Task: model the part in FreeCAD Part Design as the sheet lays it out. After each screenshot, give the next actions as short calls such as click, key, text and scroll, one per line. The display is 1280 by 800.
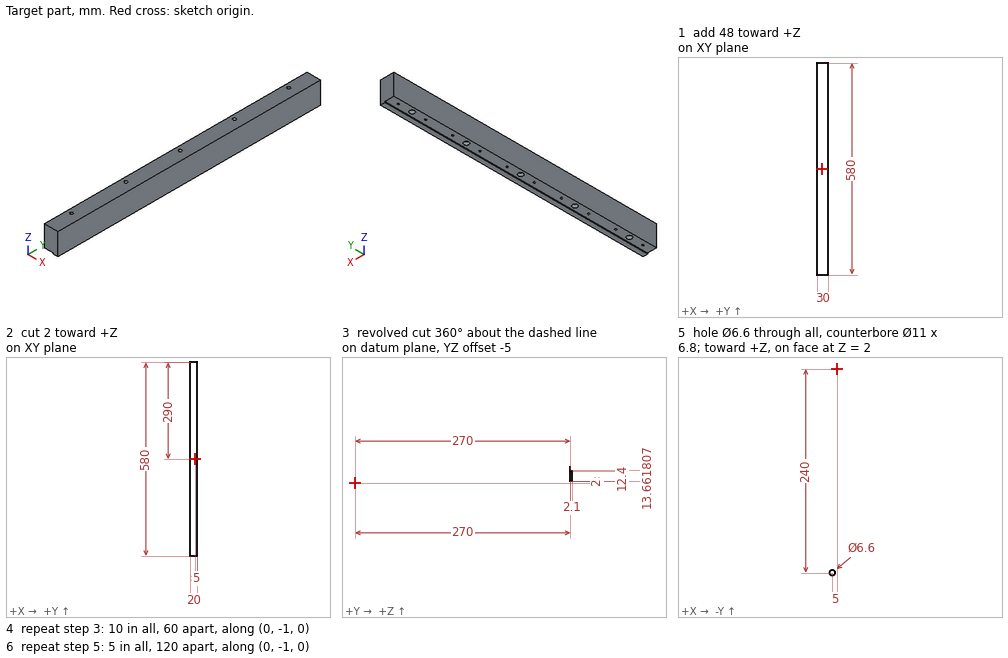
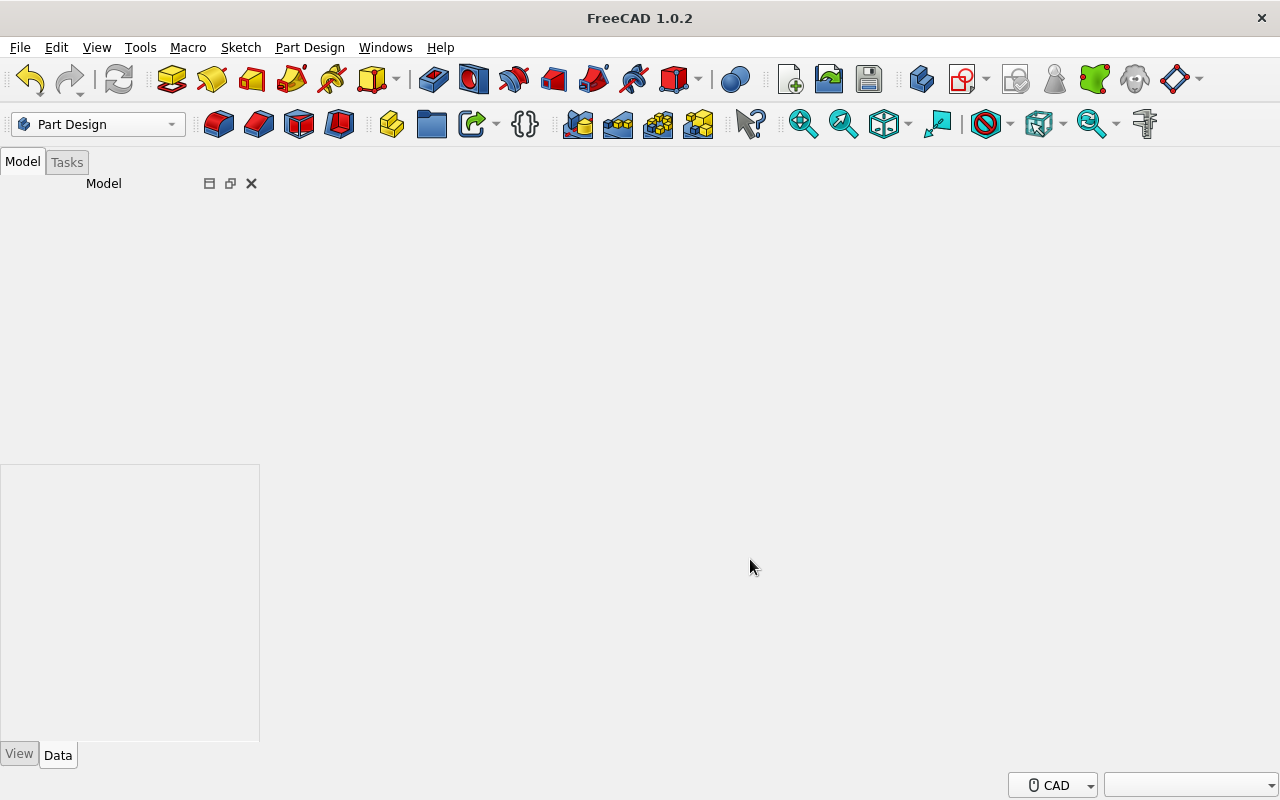
key(ctrl+n)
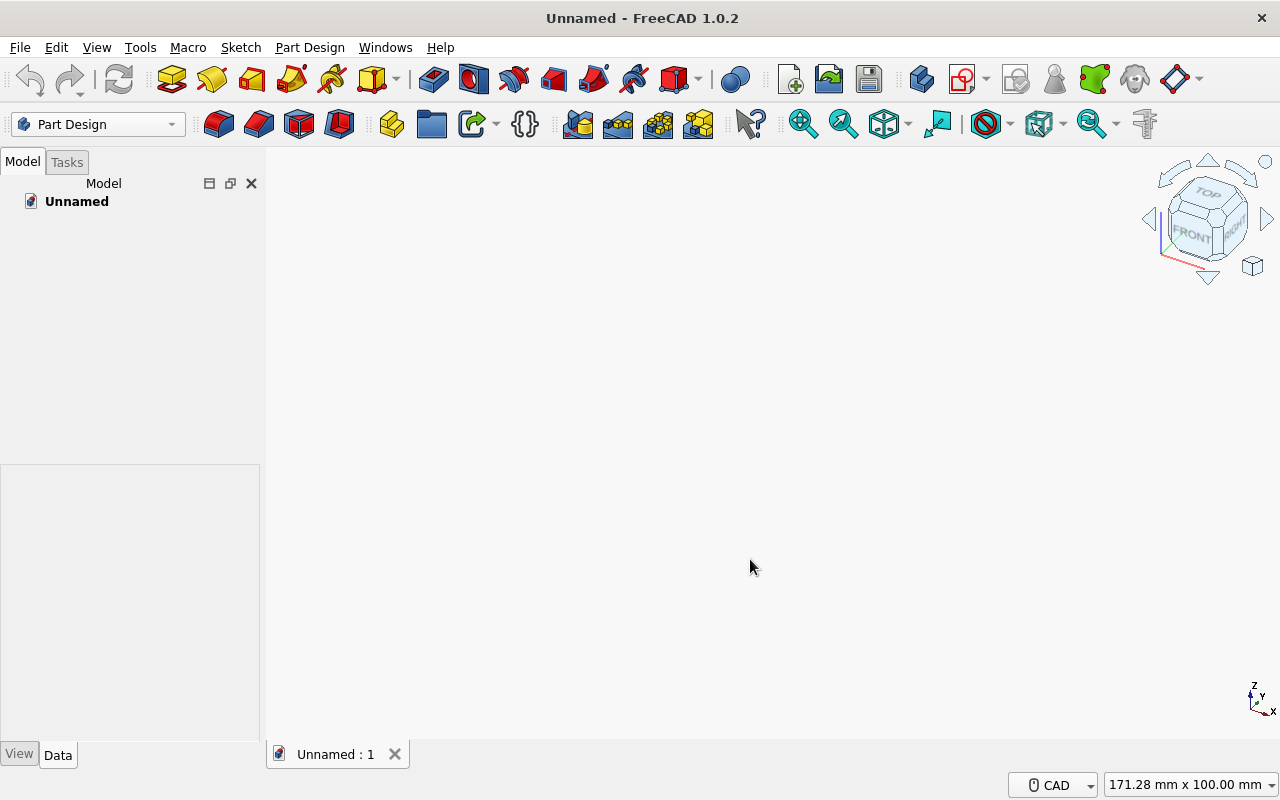
click(962, 80)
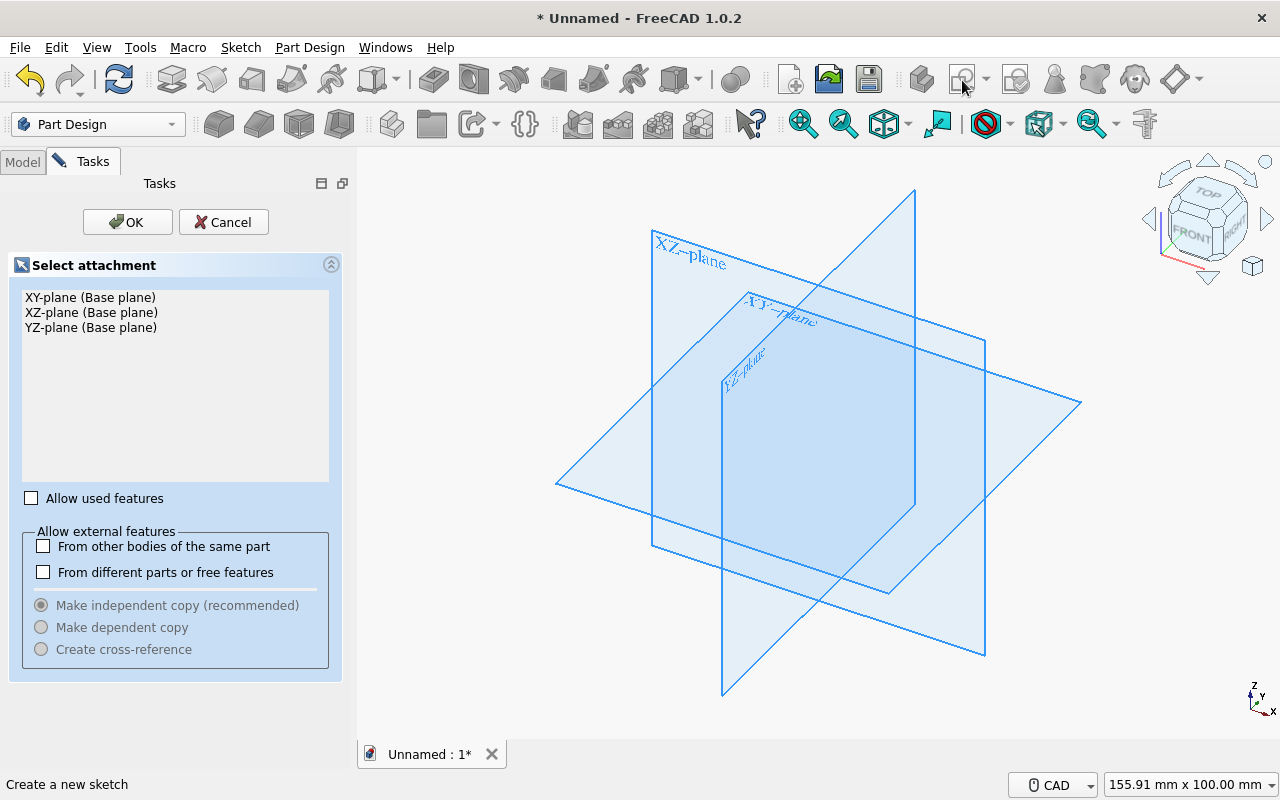
click(82, 298)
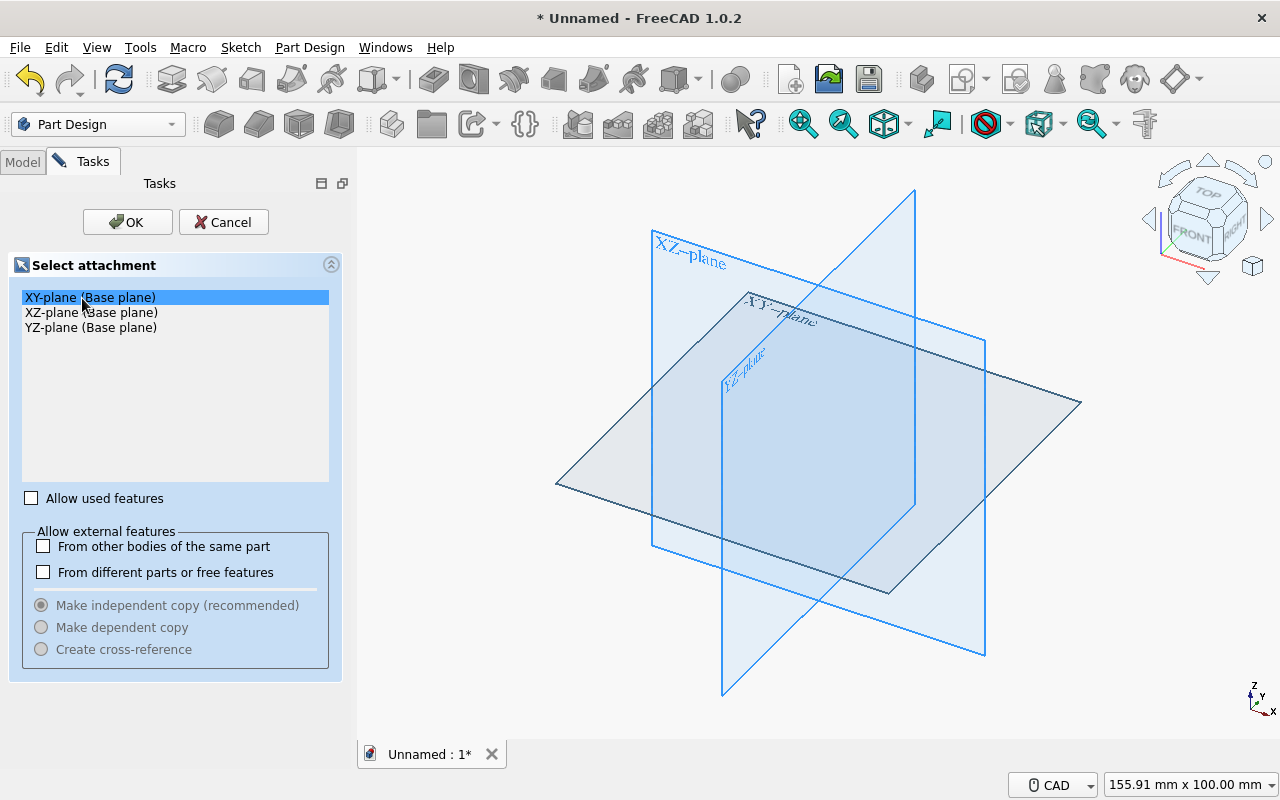
click(128, 222)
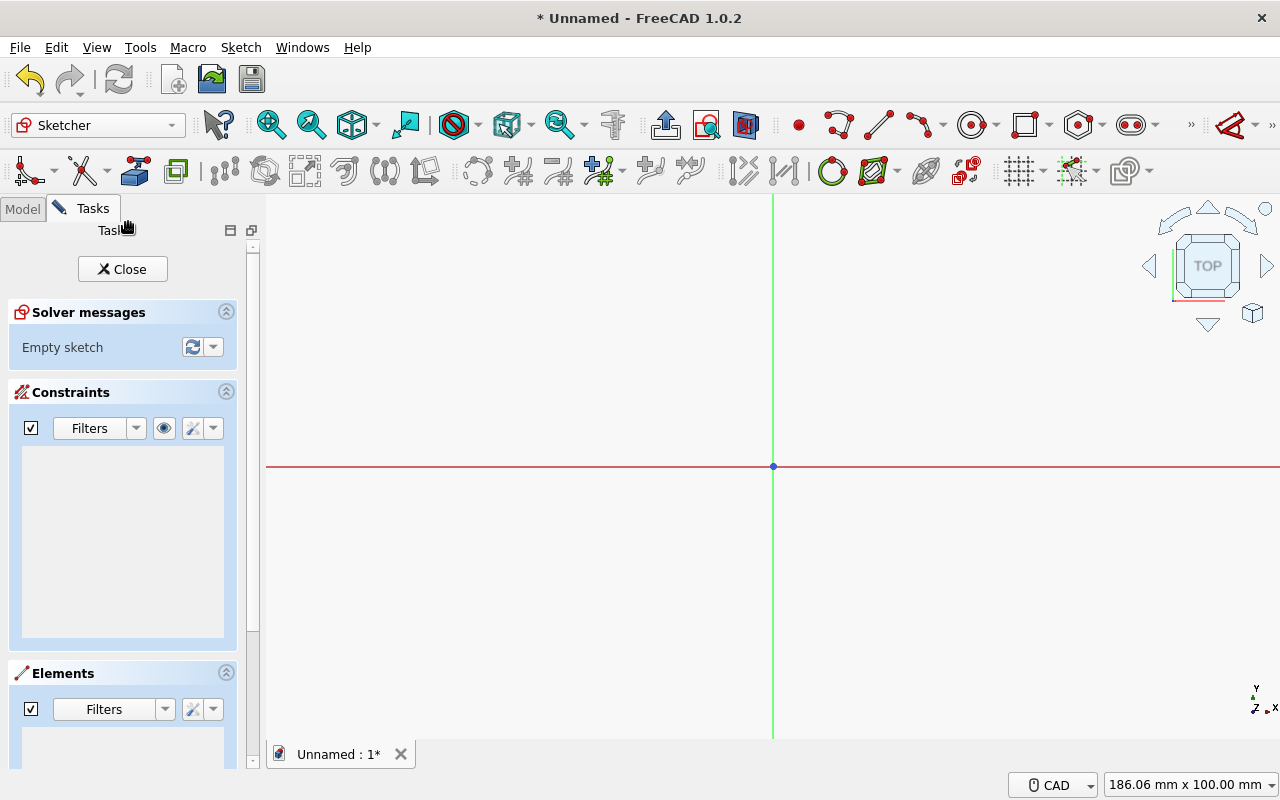
scroll(696, 467, down, 11)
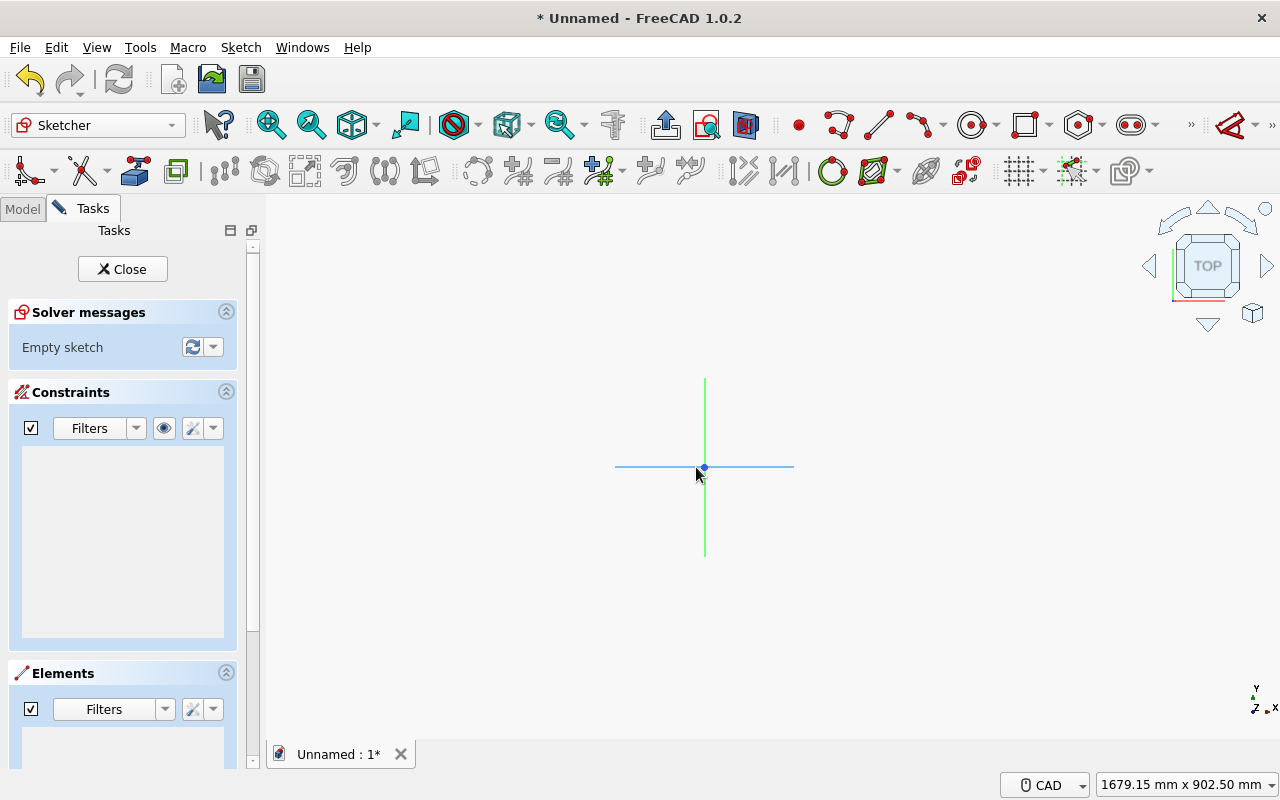
key(g)
key(v)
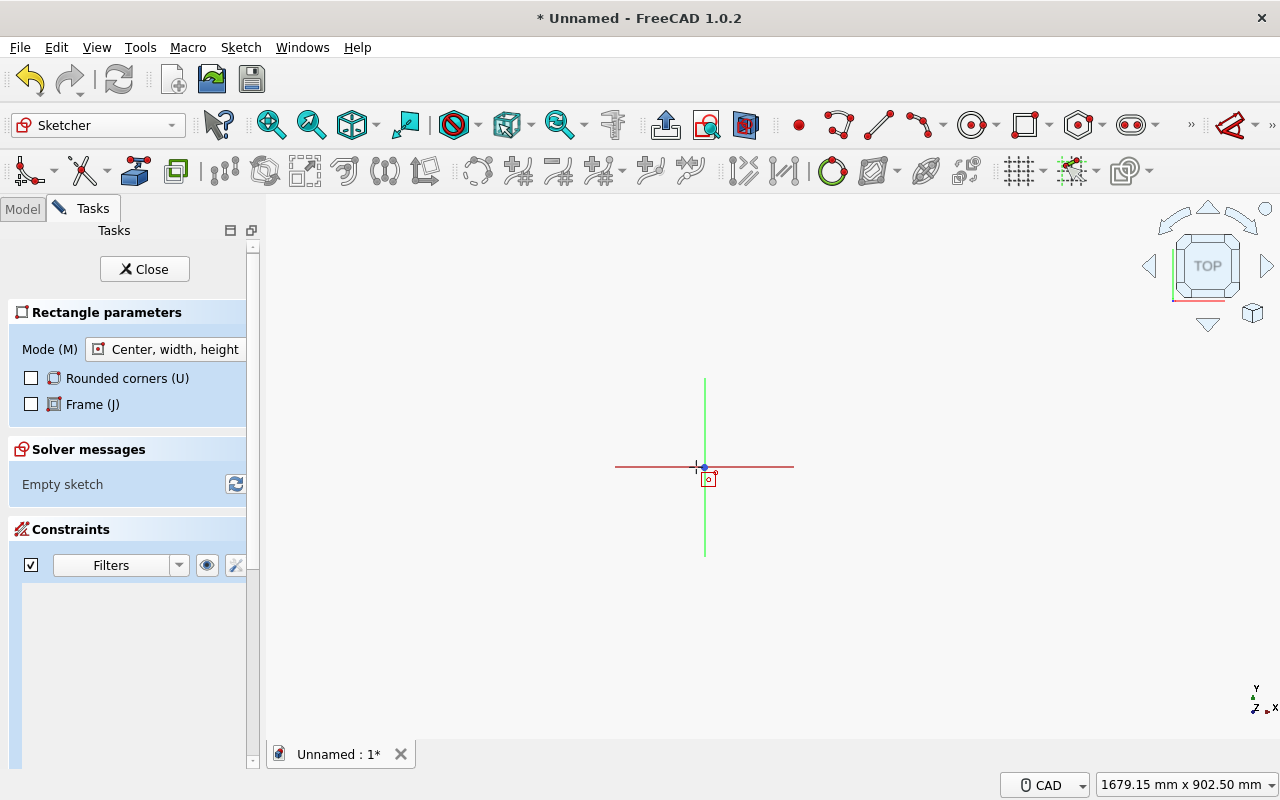
scroll(705, 467, up, 3)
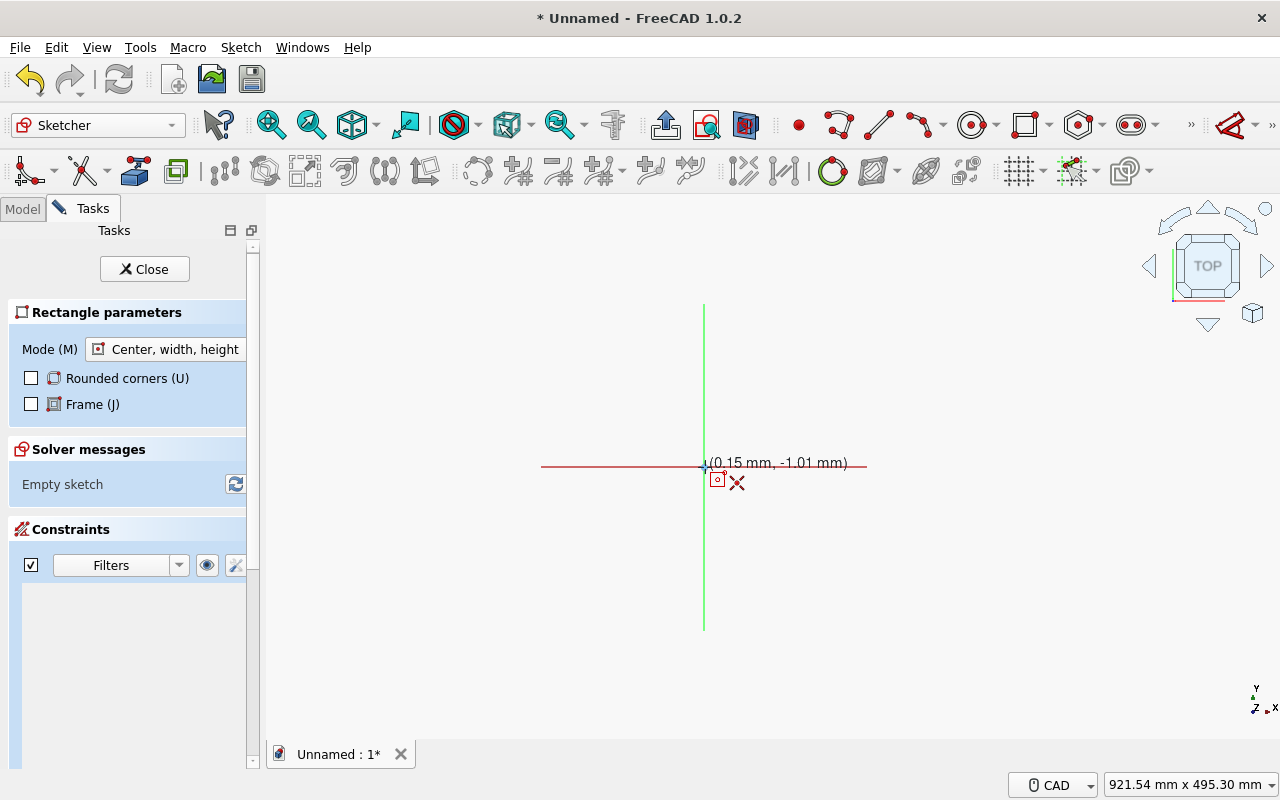
click(704, 467)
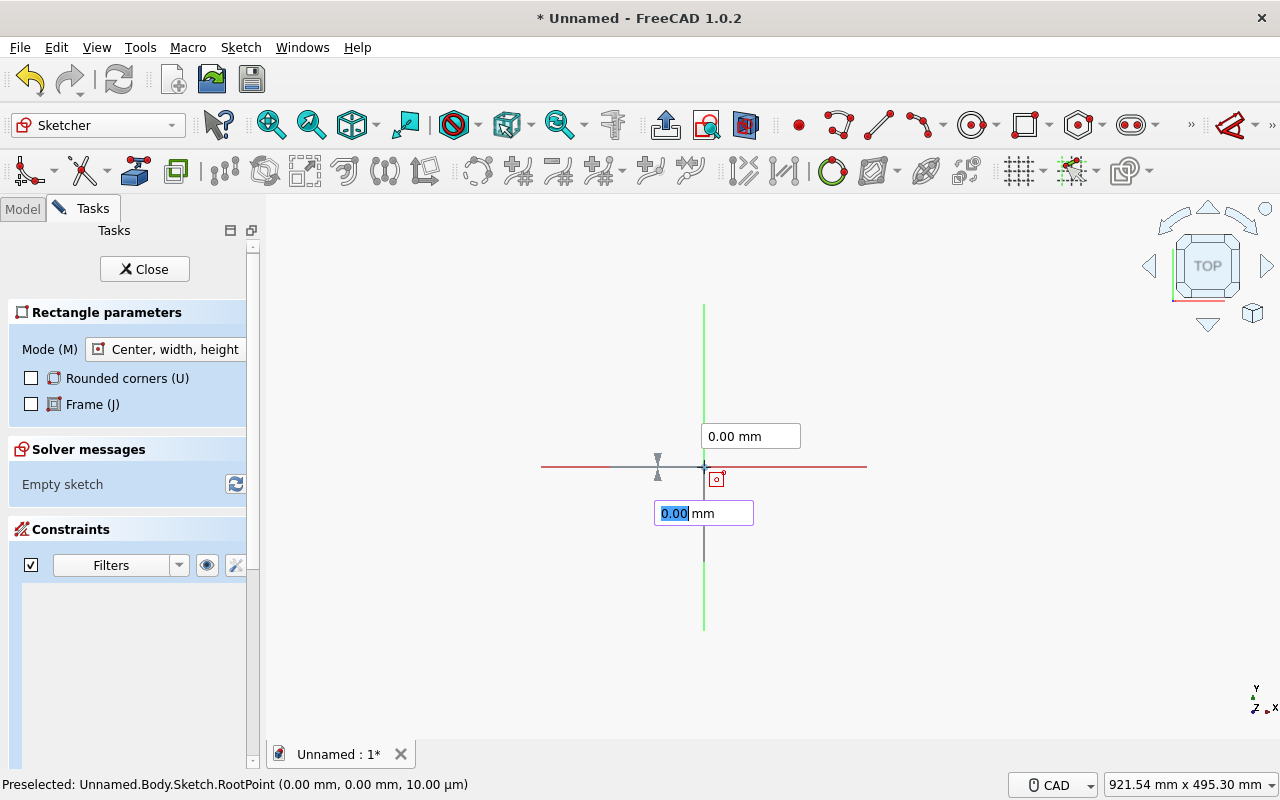
scroll(705, 466, down, 3)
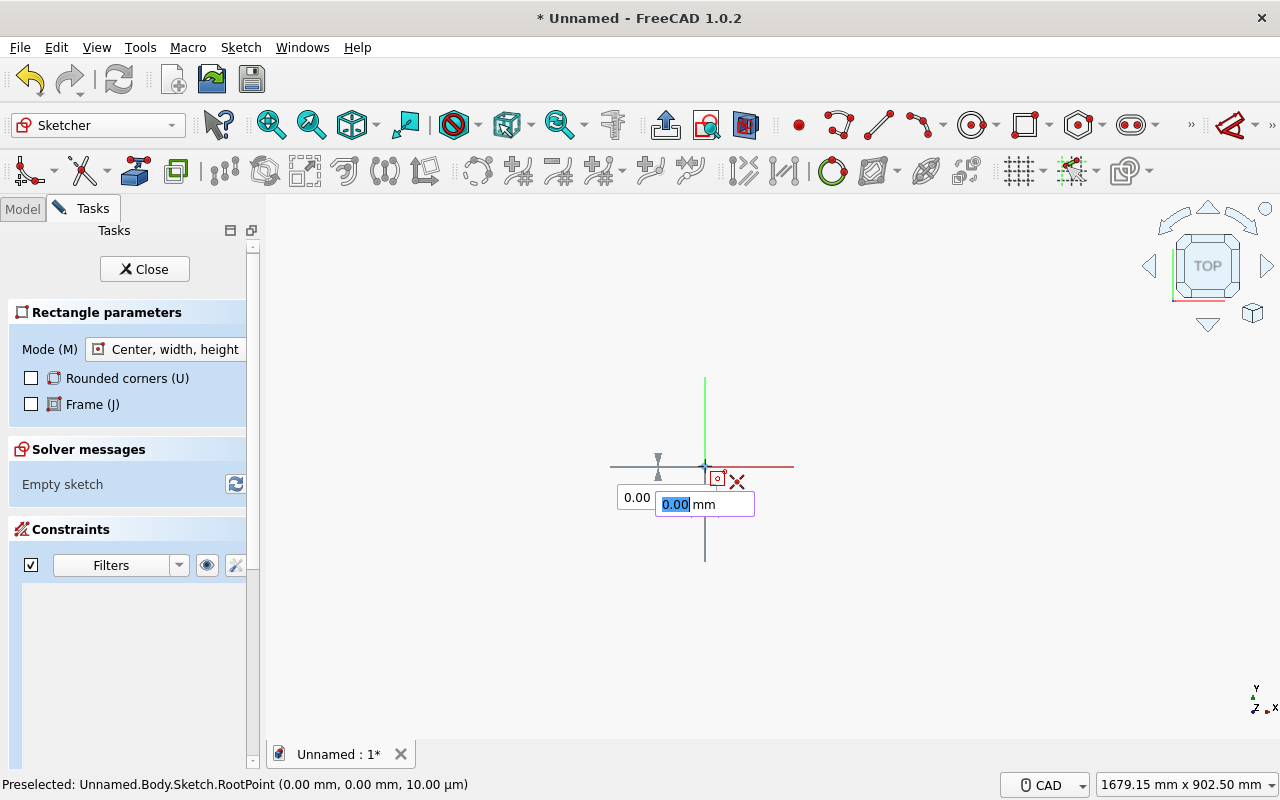
scroll(714, 292, up, 3)